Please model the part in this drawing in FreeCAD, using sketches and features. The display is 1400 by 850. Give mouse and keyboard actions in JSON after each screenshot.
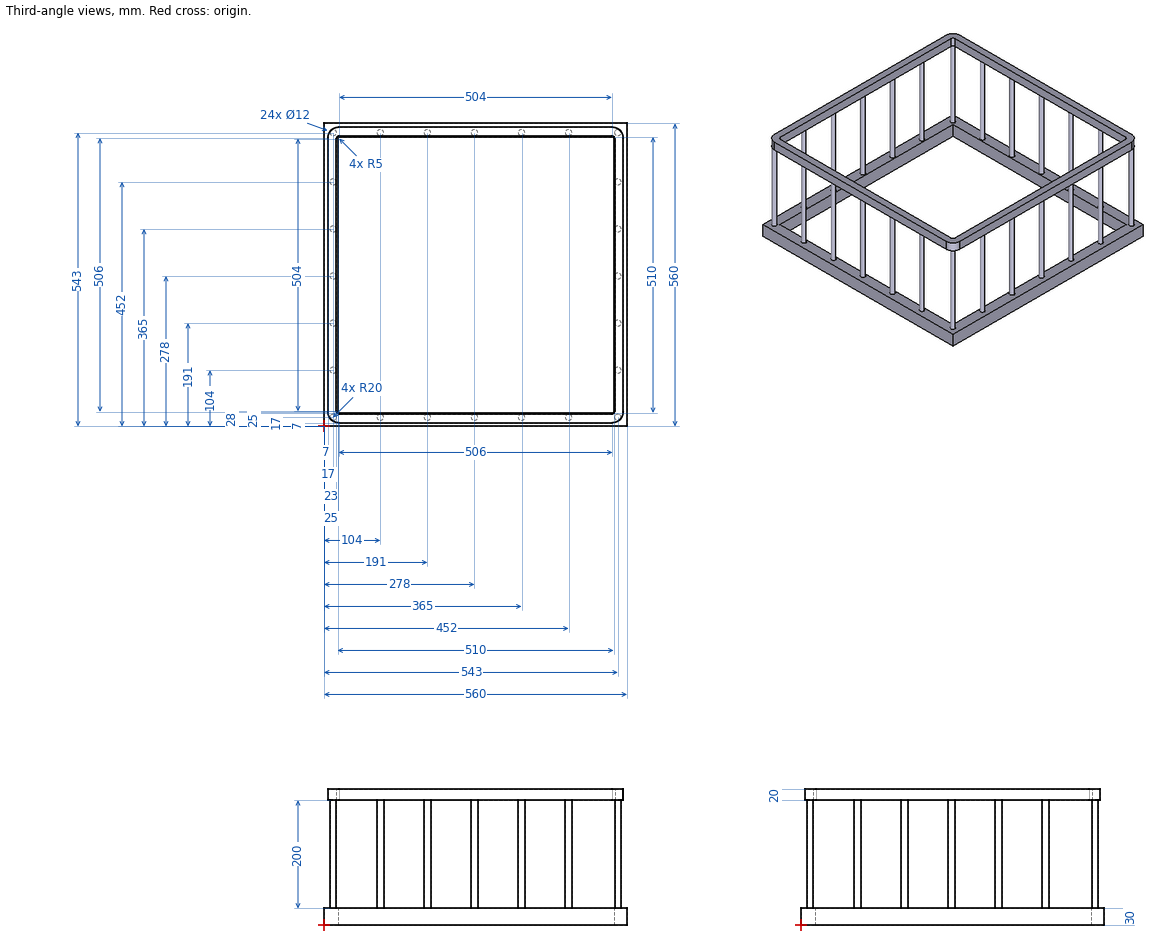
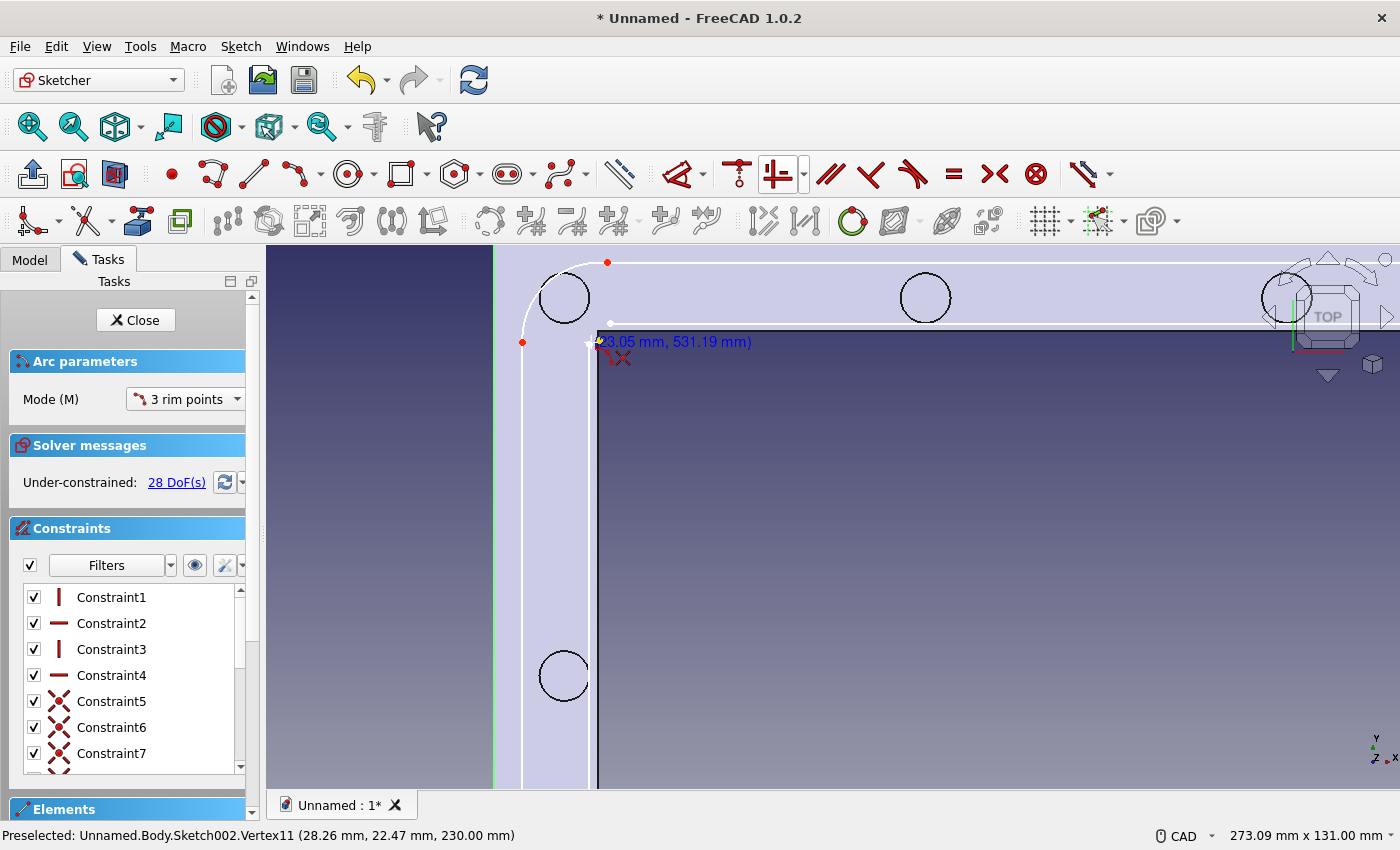
{"action": "left_click", "coordinate": [589, 345]}
{"action": "left_click", "coordinate": [610, 324]}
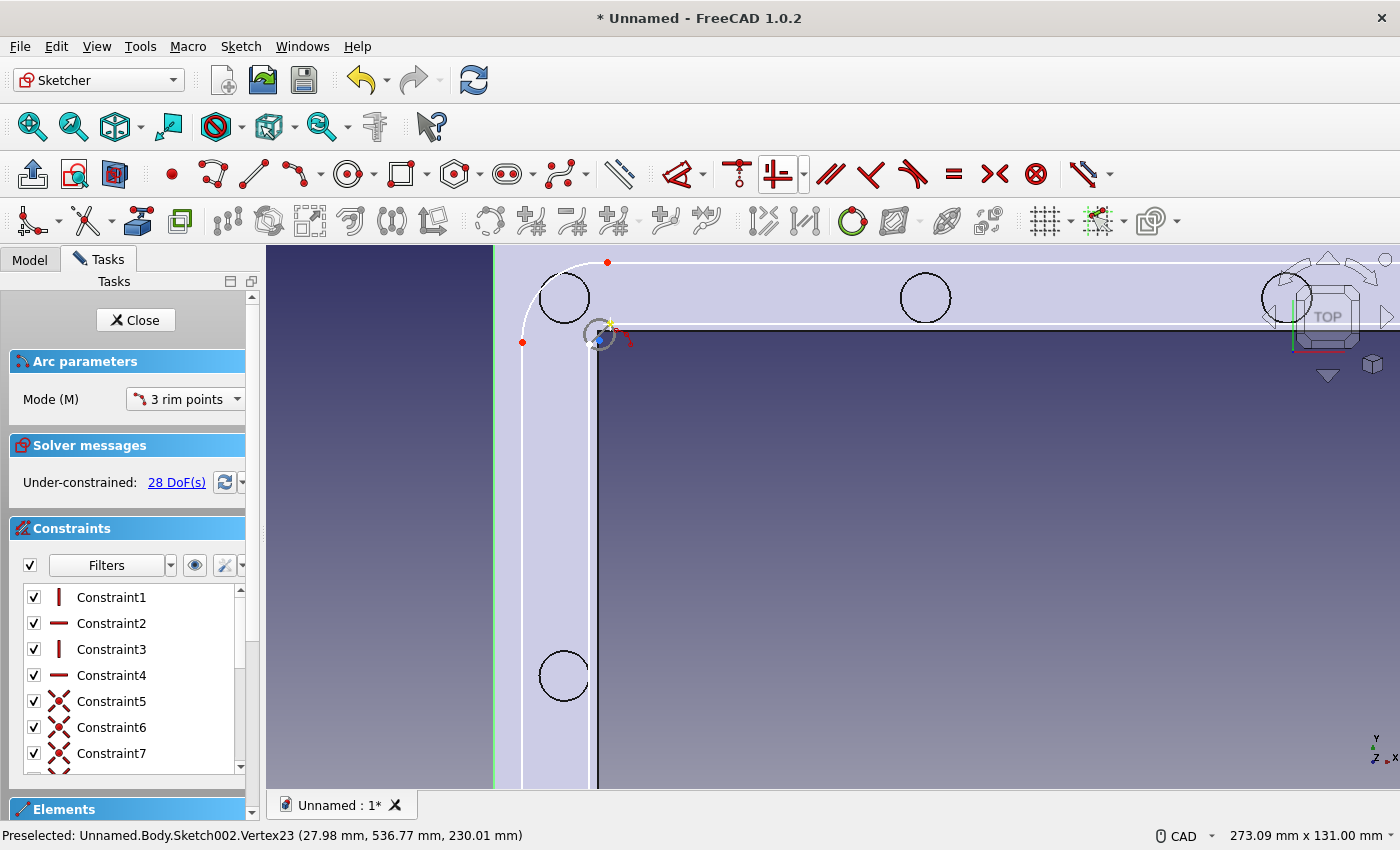
{"action": "scroll", "coordinate": [595, 329], "scroll_direction": "up", "scroll_amount": 5}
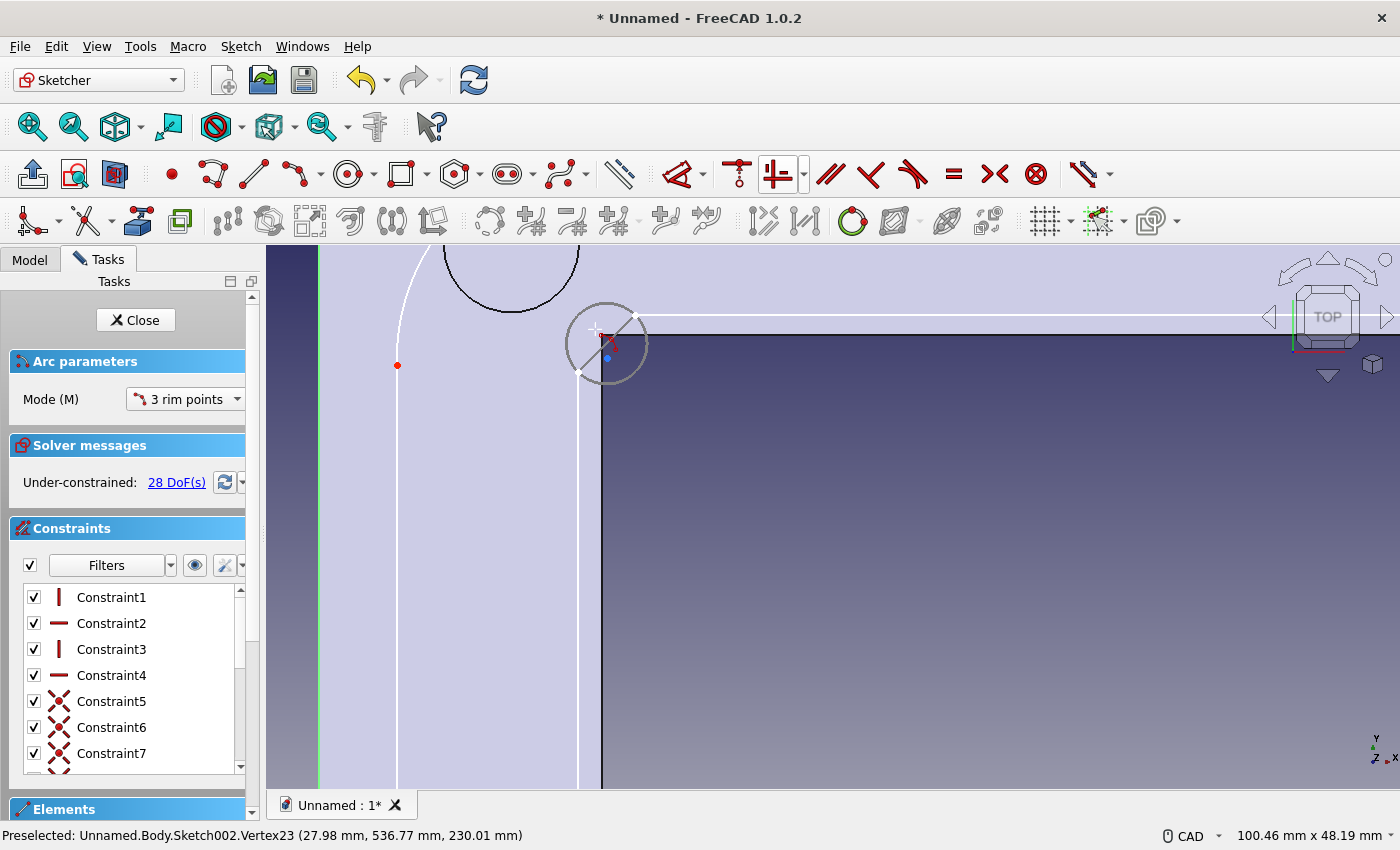
{"action": "left_click", "coordinate": [596, 329]}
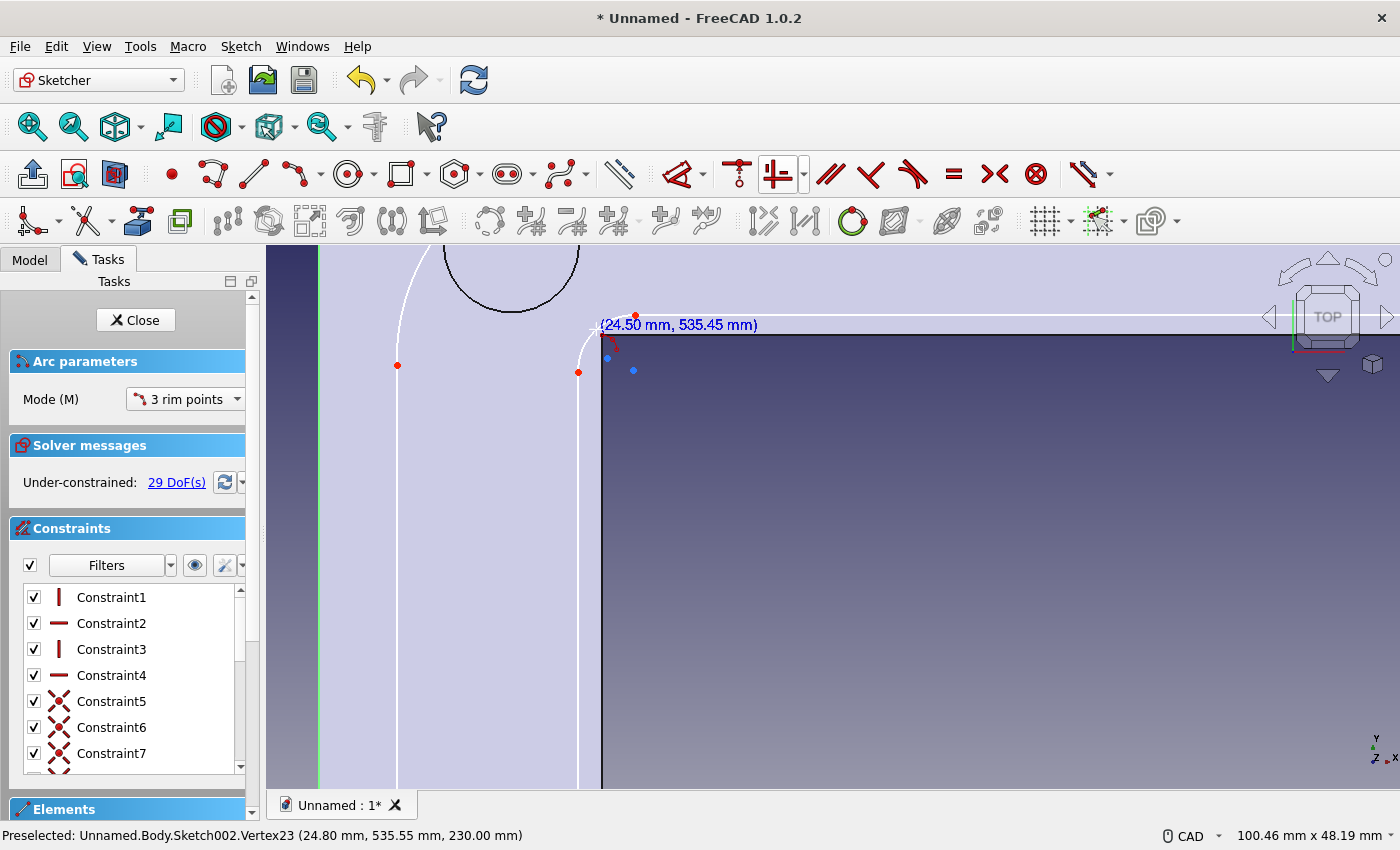
{"action": "scroll", "coordinate": [591, 340], "scroll_direction": "down", "scroll_amount": 14}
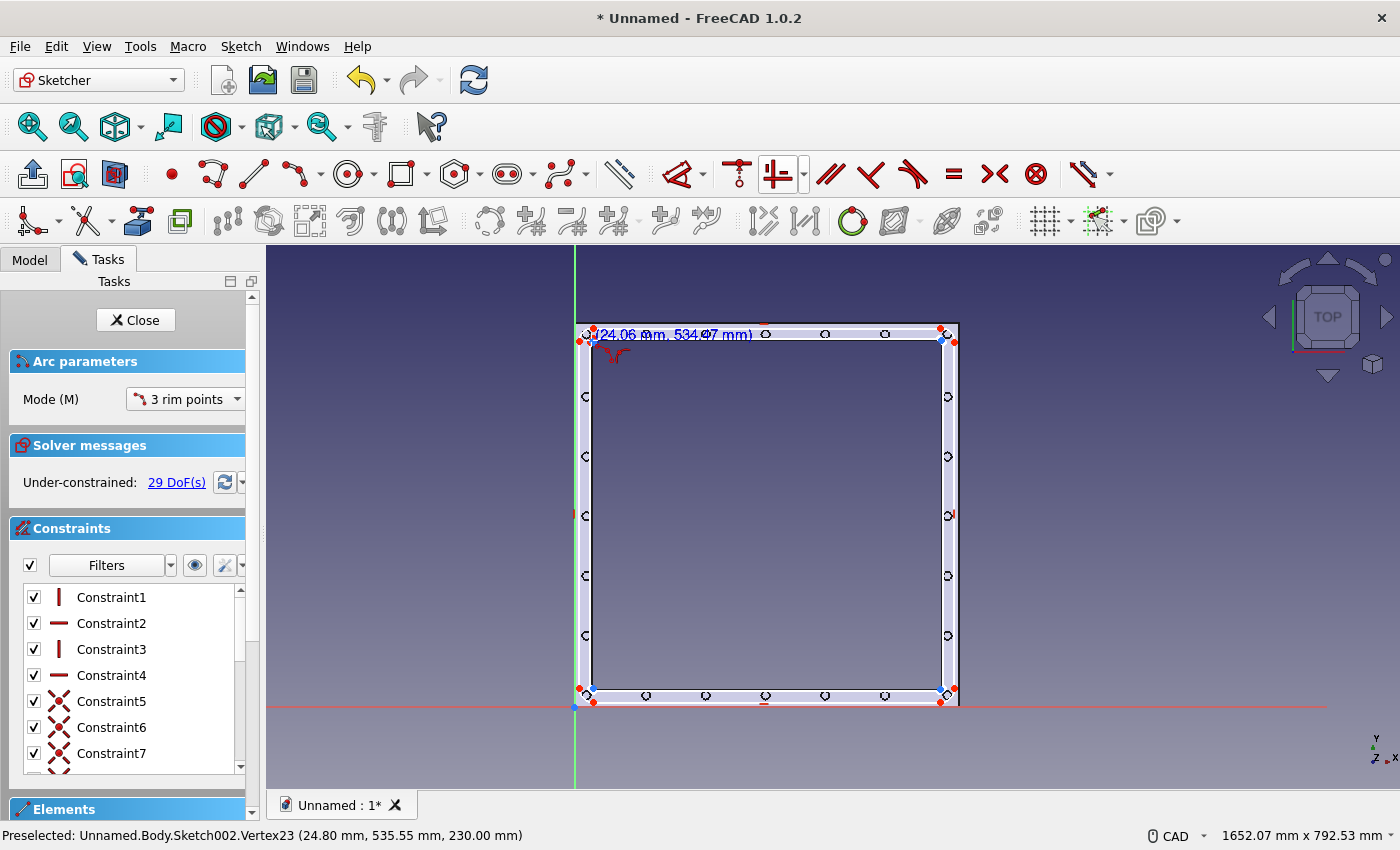
{"action": "scroll", "coordinate": [940, 338], "scroll_direction": "up", "scroll_amount": 9}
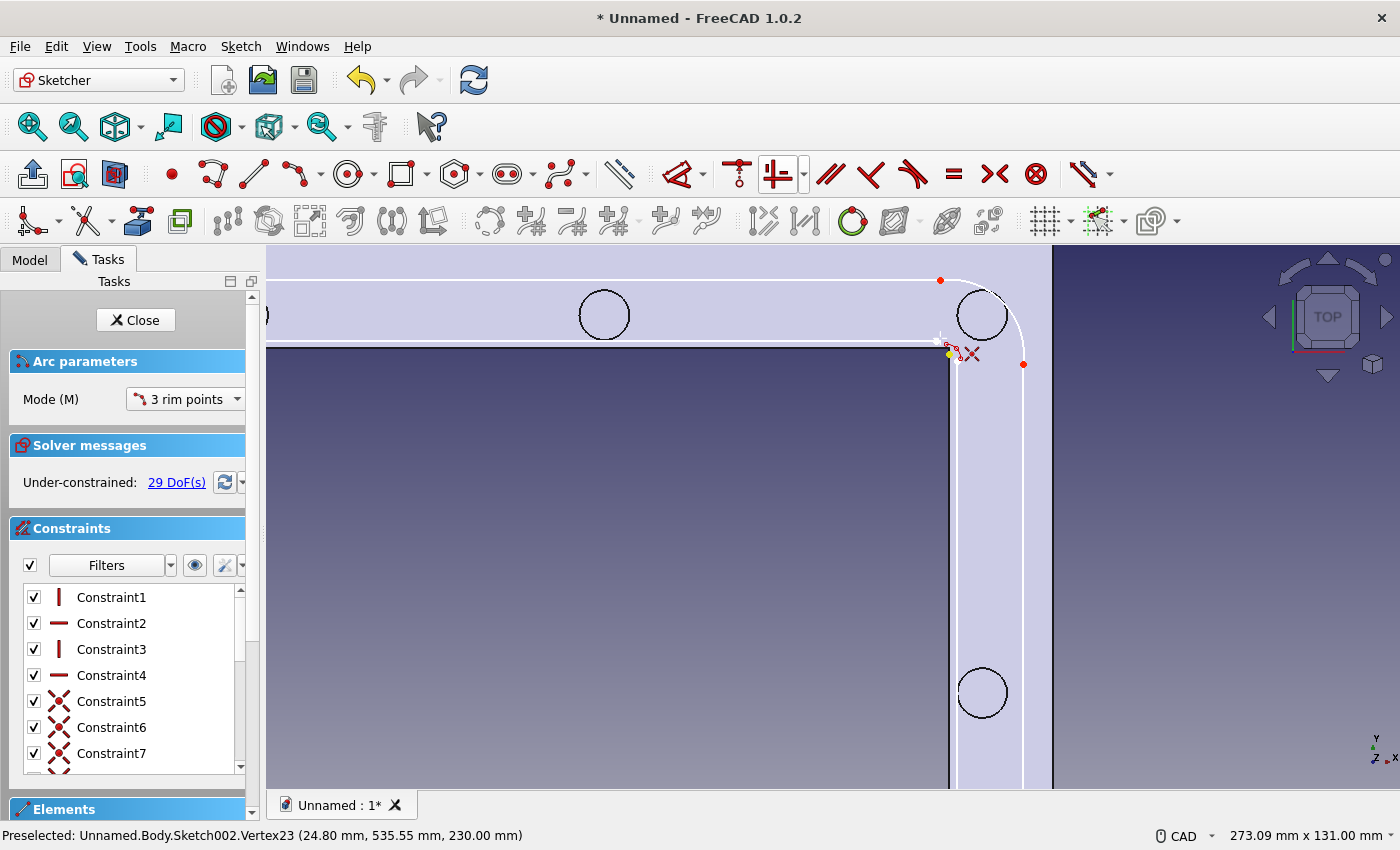
{"action": "left_click", "coordinate": [936, 341]}
{"action": "left_click", "coordinate": [957, 362]}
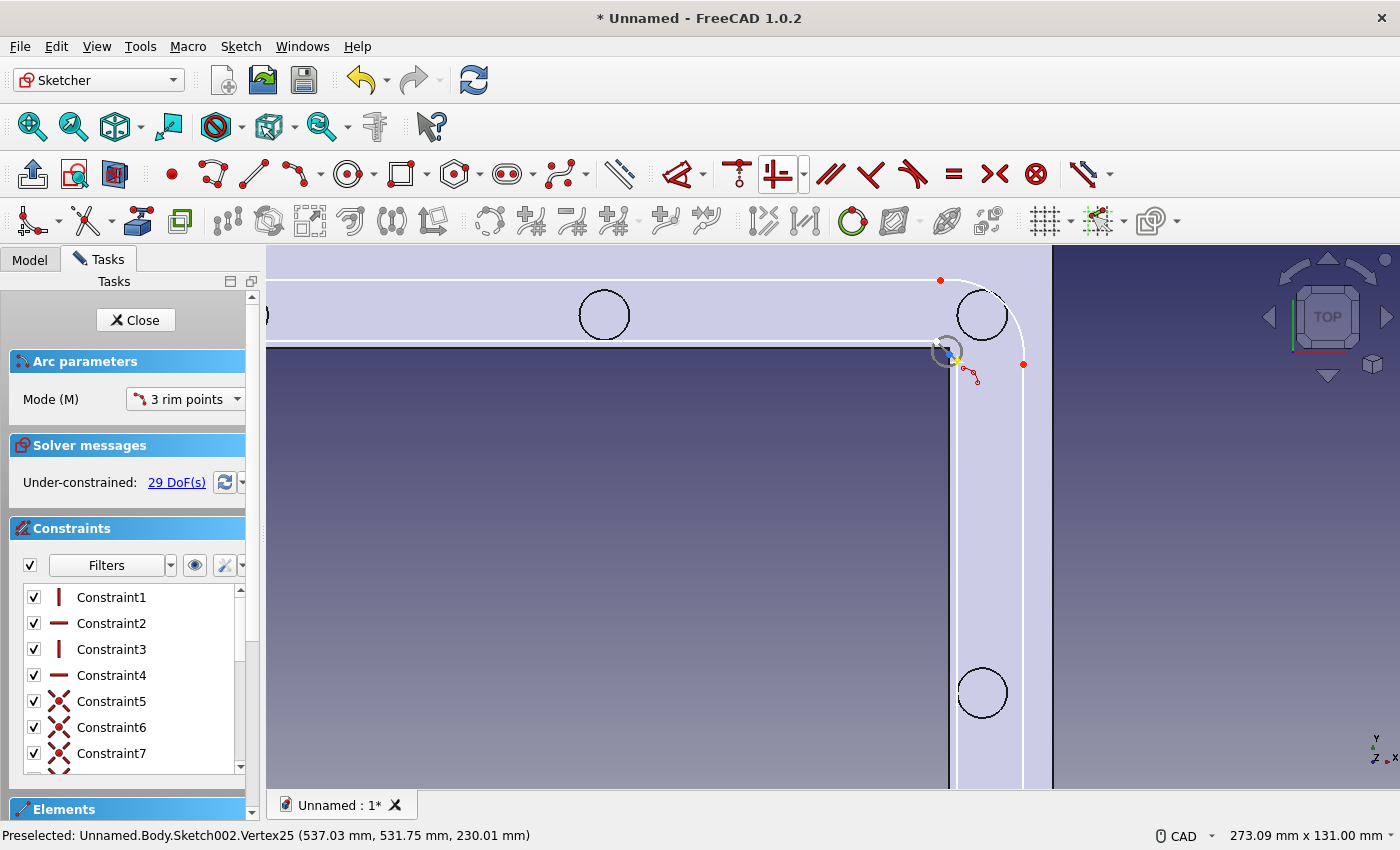
{"action": "scroll", "coordinate": [951, 346], "scroll_direction": "up", "scroll_amount": 5}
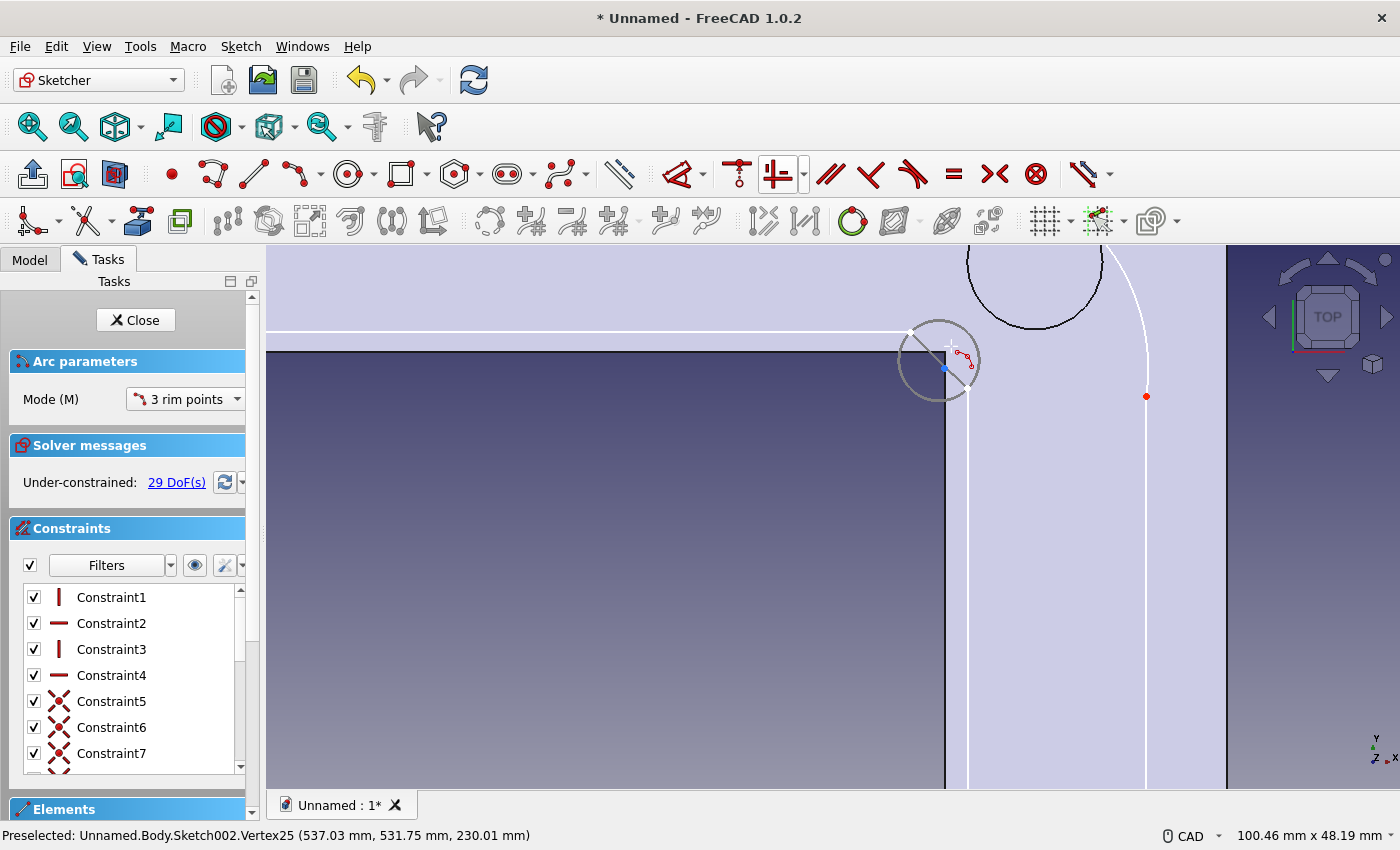
{"action": "left_click", "coordinate": [951, 346]}